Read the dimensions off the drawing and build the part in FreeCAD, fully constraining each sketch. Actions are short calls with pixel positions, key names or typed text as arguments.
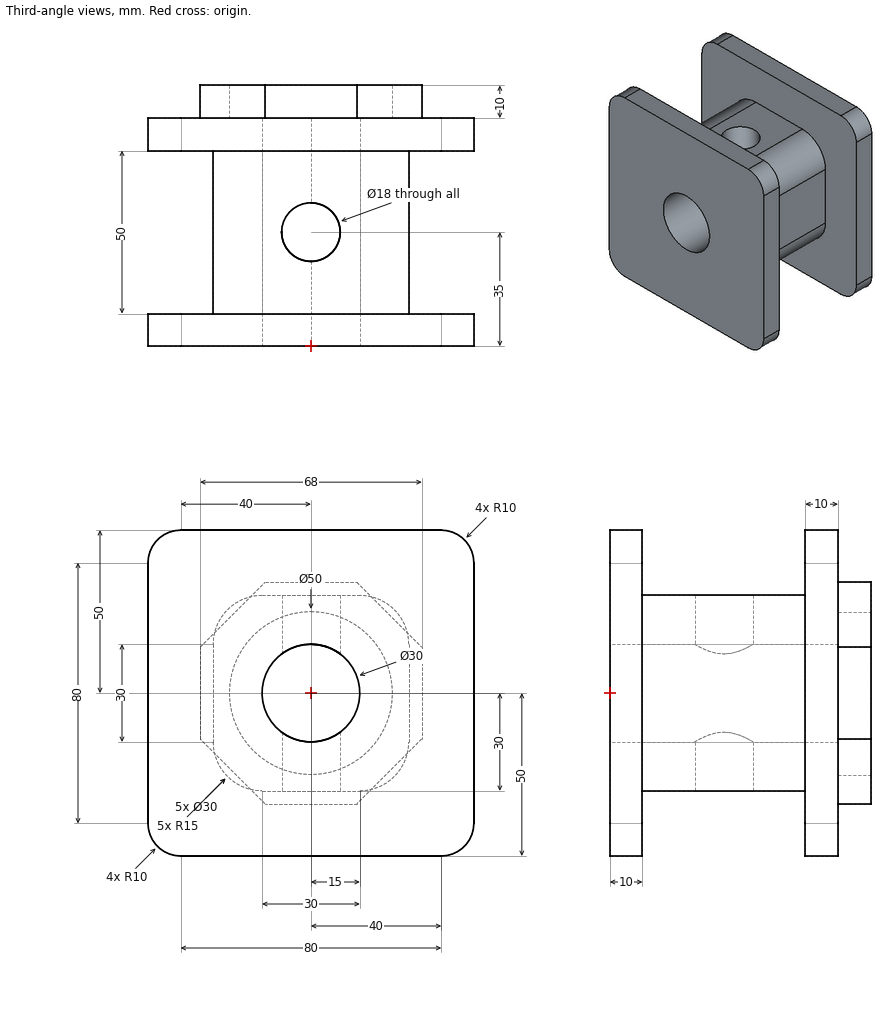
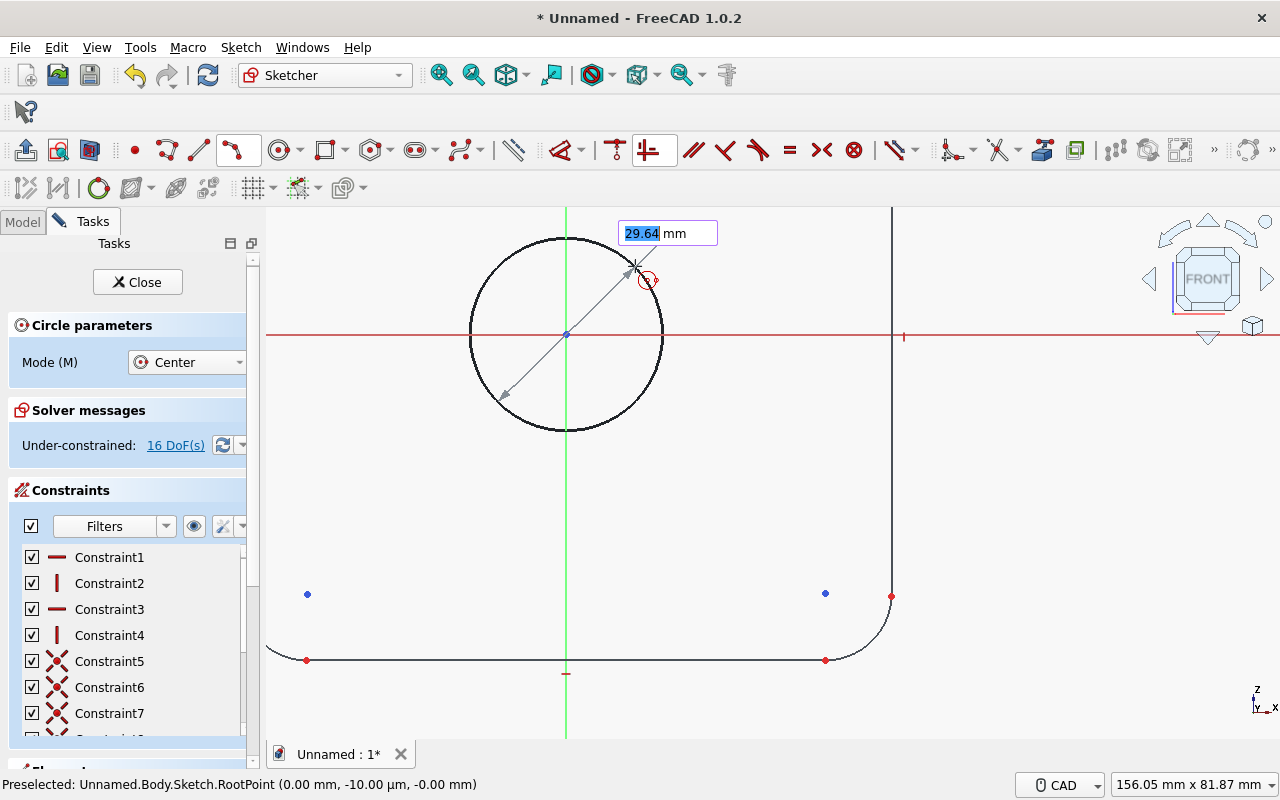
text(30)
key(Return)
key(Escape)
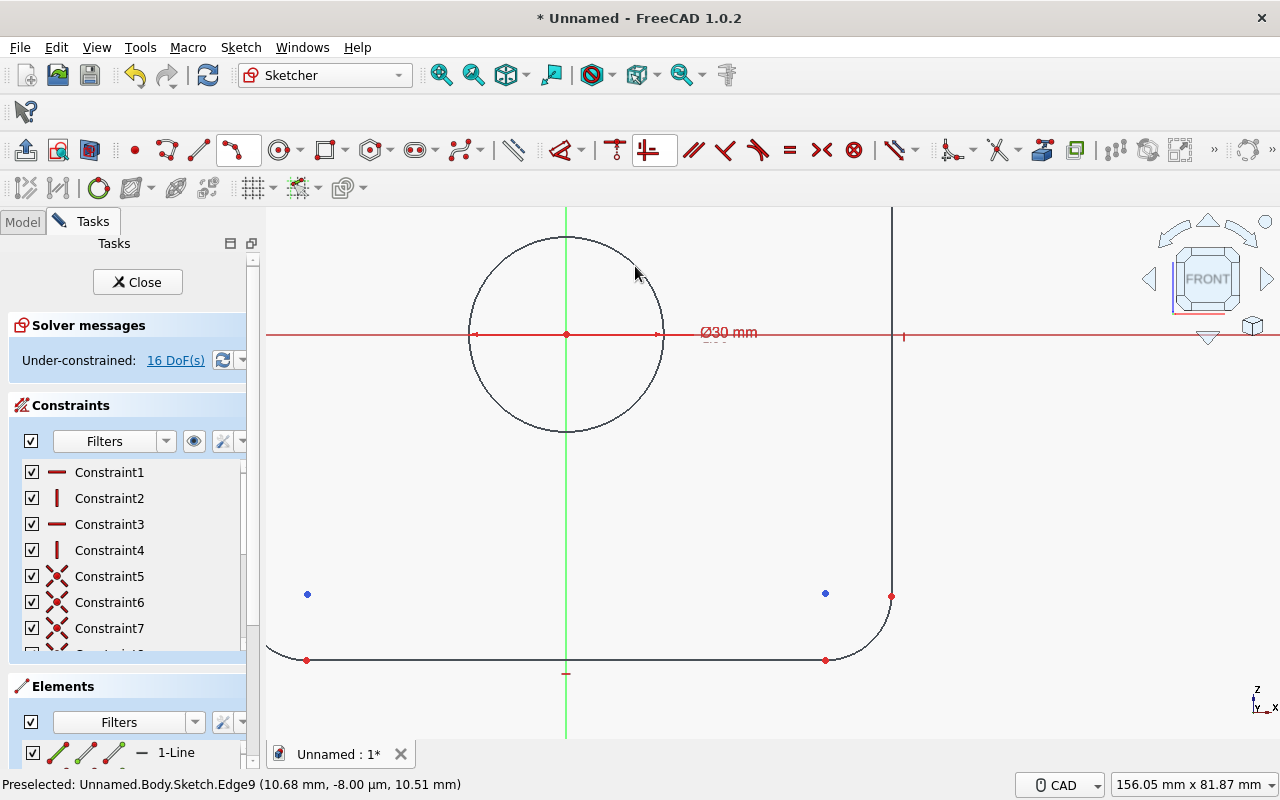
click(670, 660)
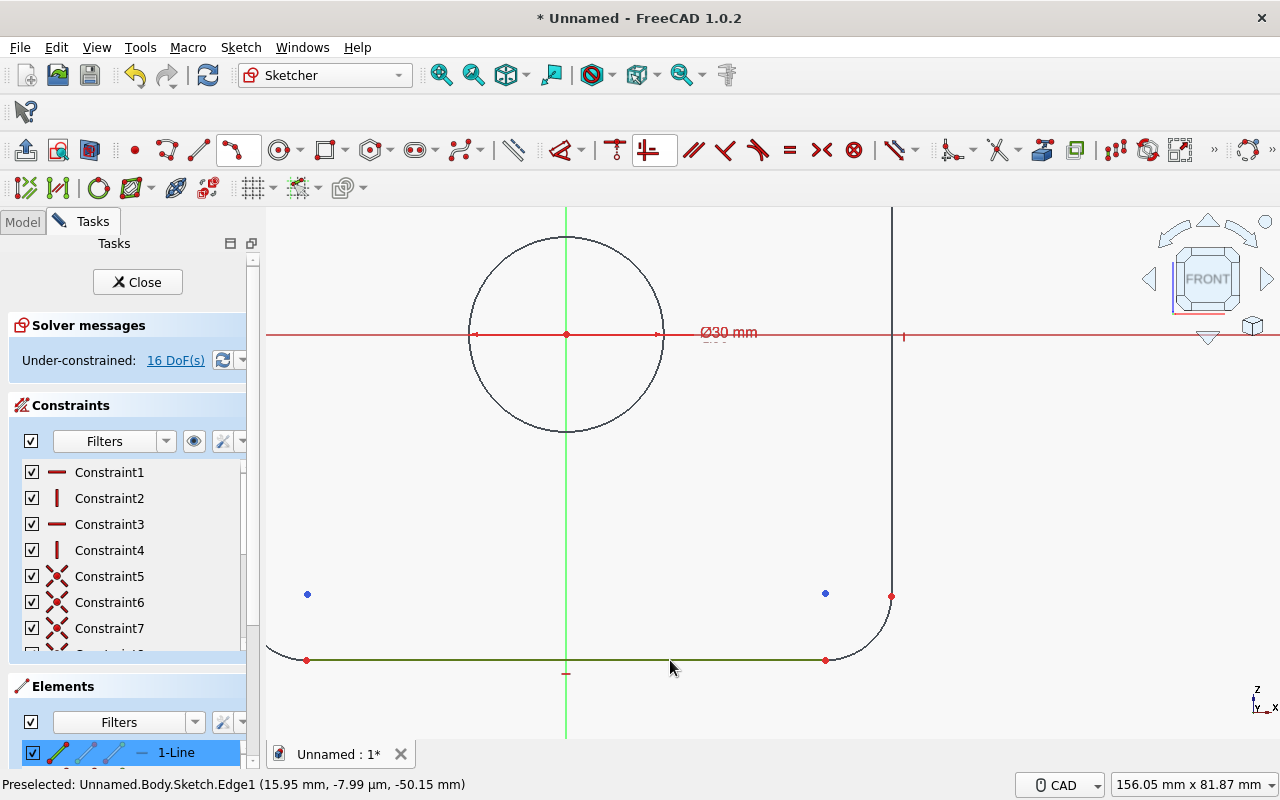
scroll(873, 641, down, 3)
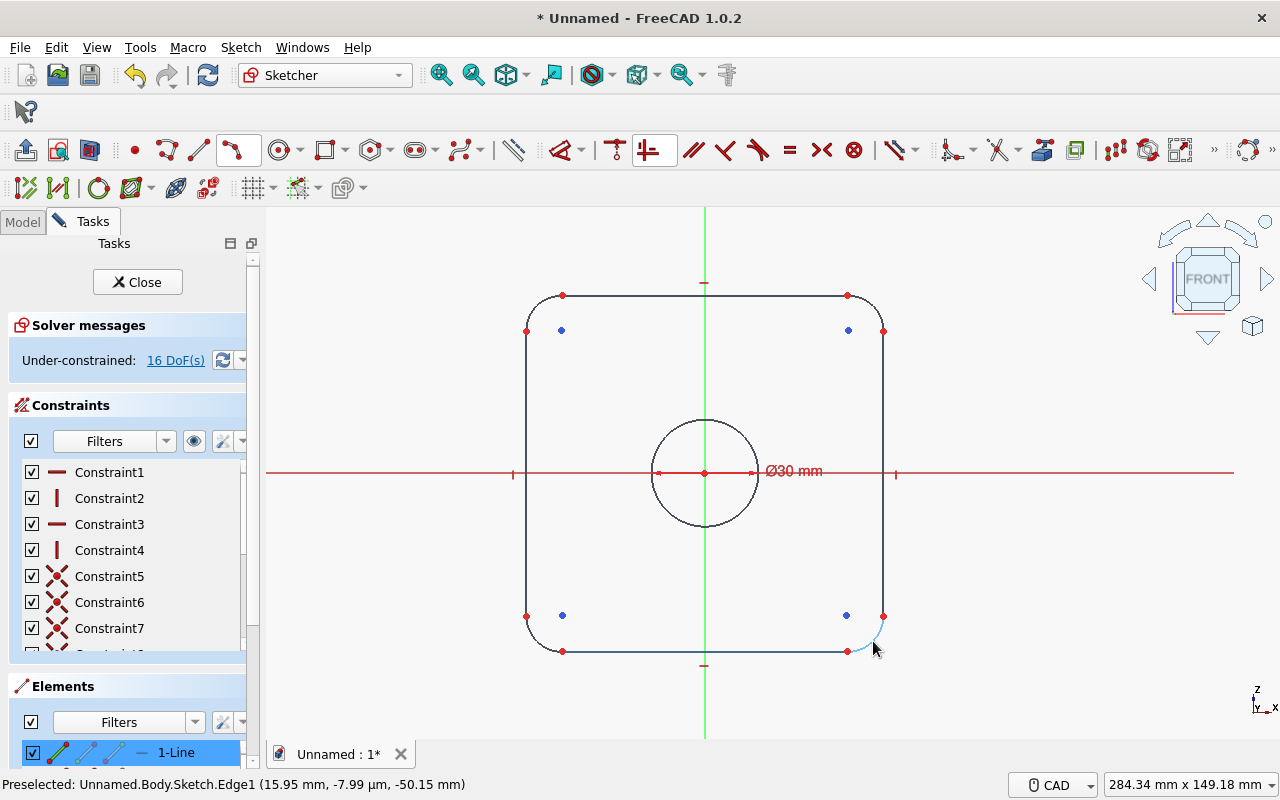
click(531, 633)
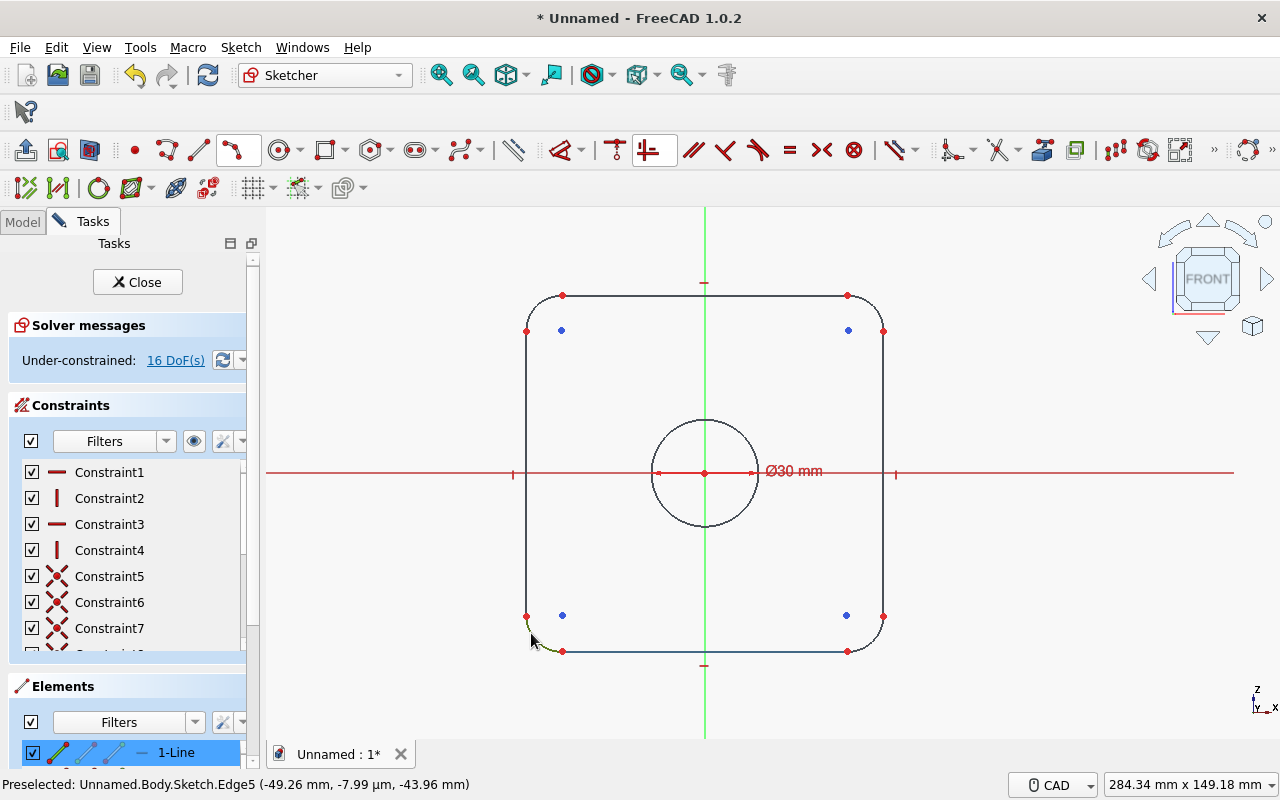
click(758, 150)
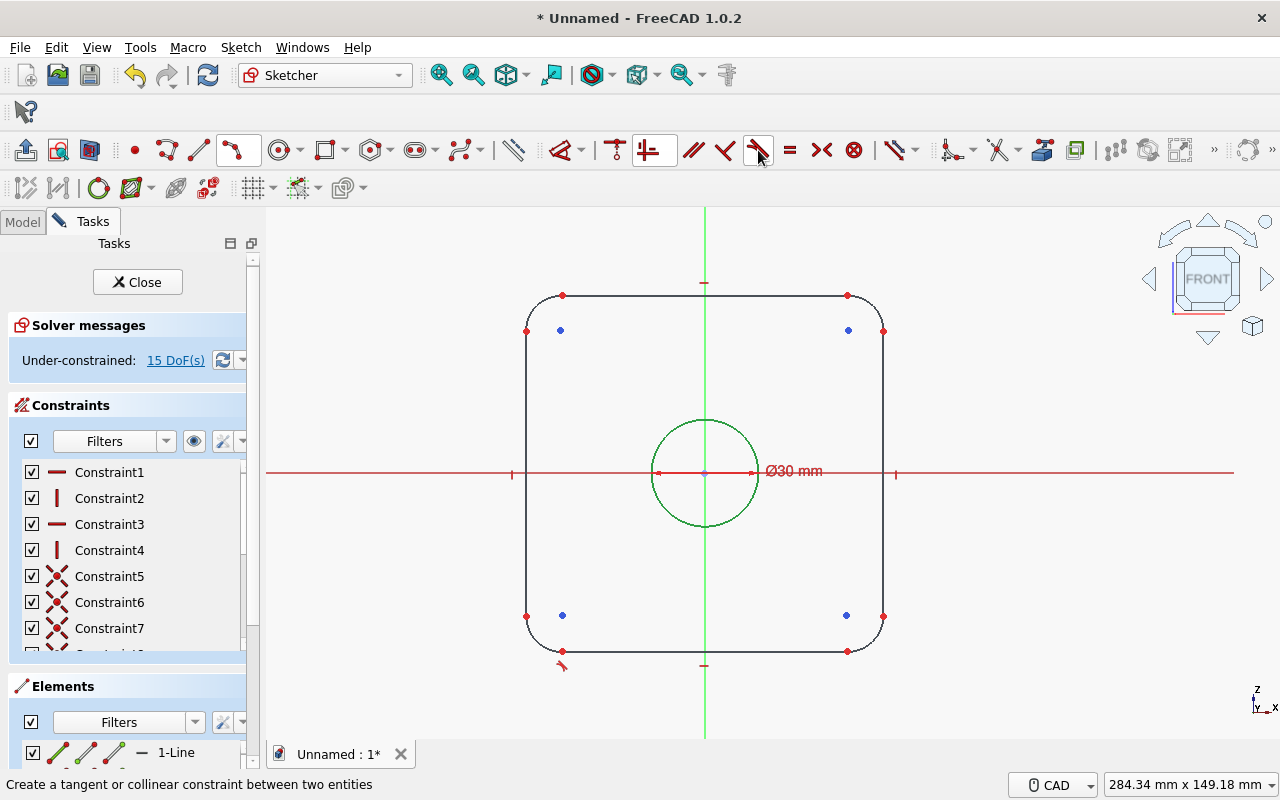
click(762, 652)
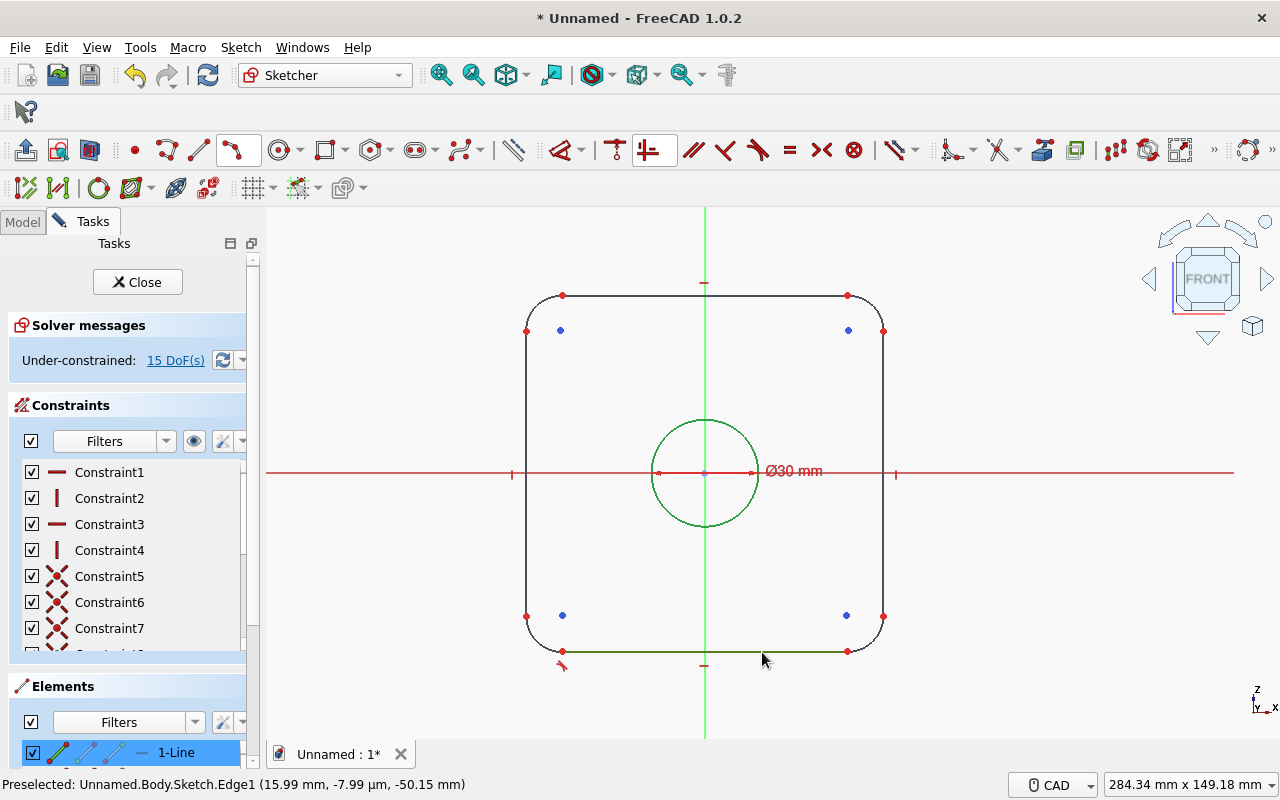
click(863, 648)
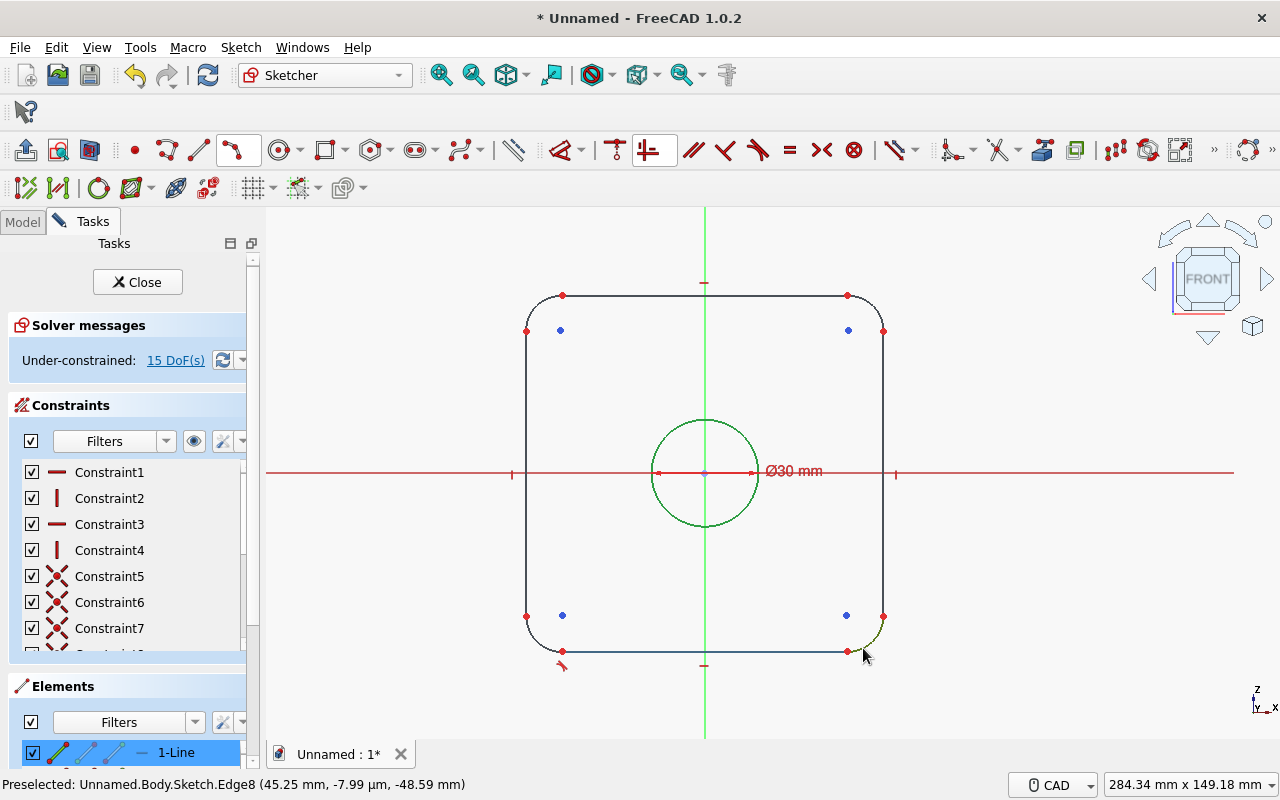
click(758, 150)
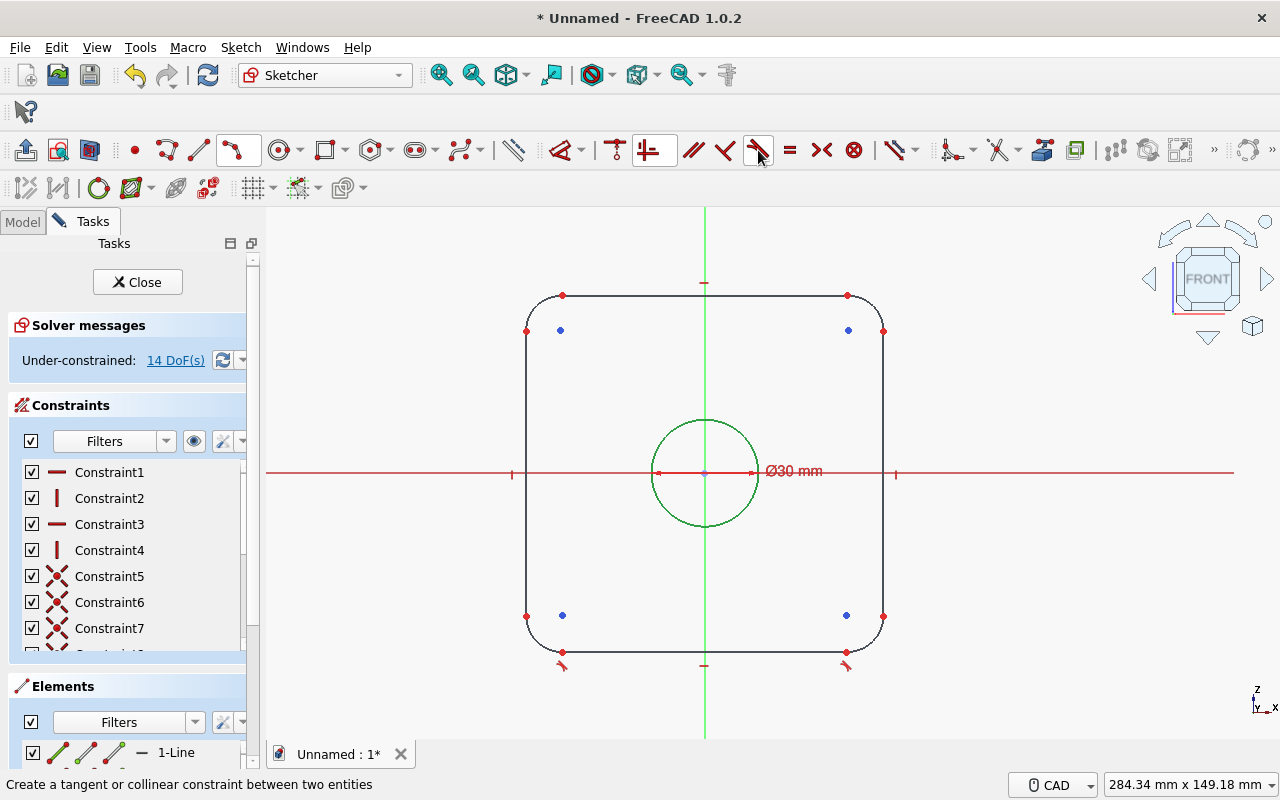
click(526, 532)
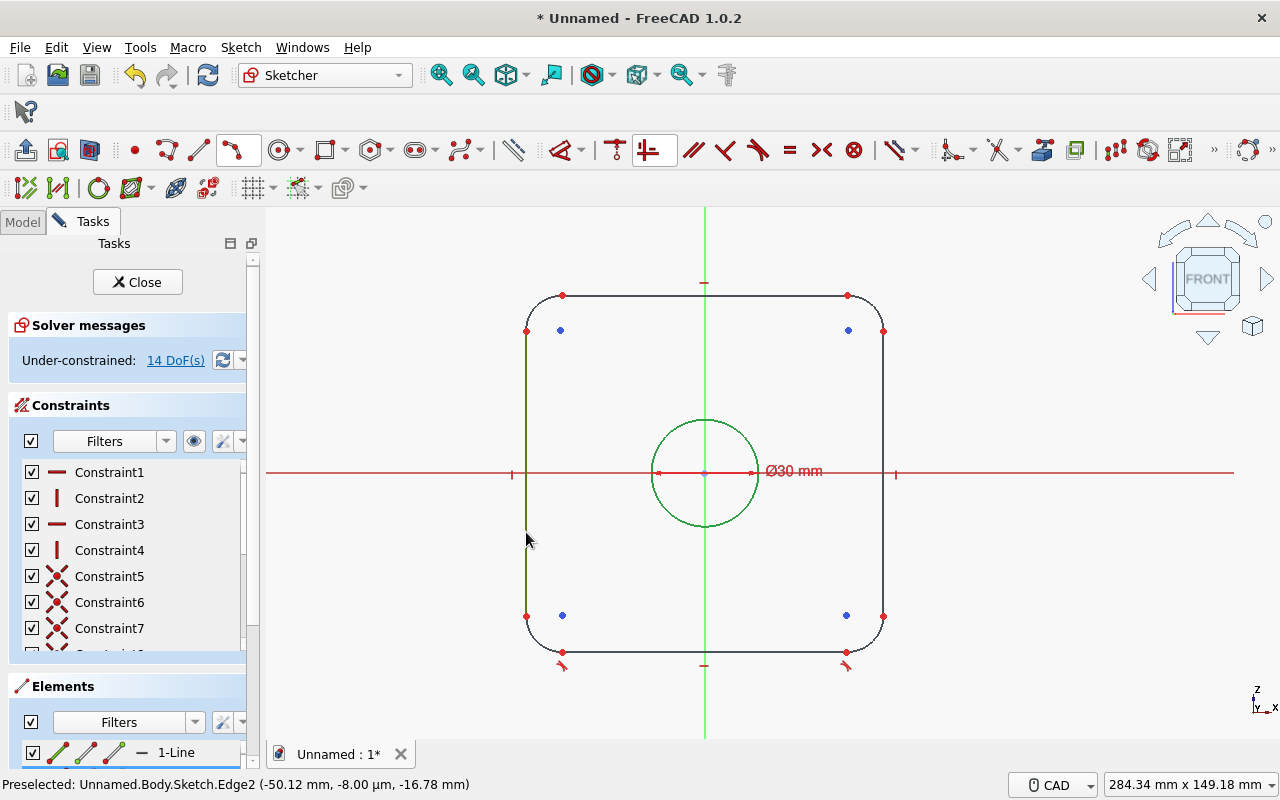
click(531, 633)